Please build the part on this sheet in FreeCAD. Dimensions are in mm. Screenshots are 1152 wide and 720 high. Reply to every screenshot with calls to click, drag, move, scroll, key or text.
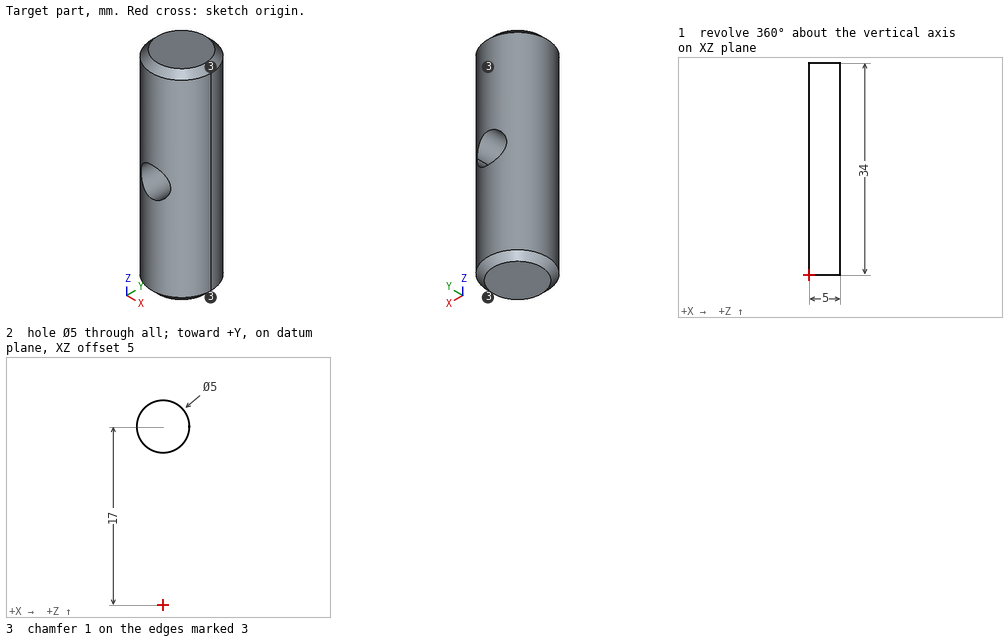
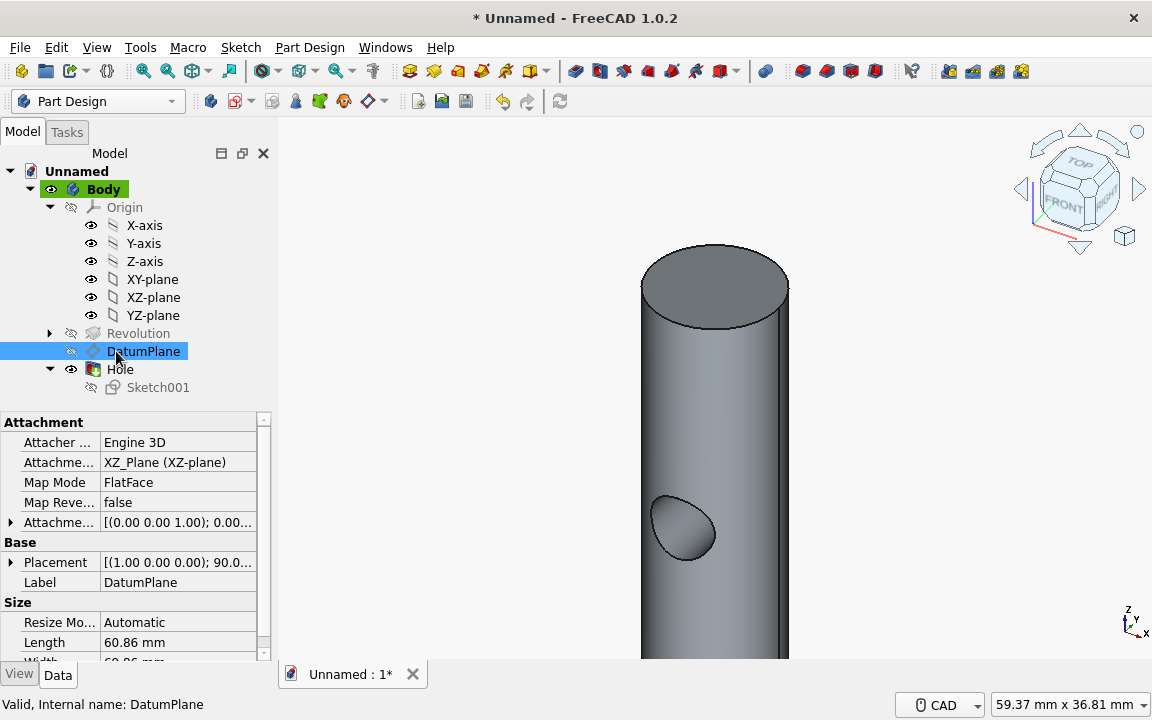
click(144, 72)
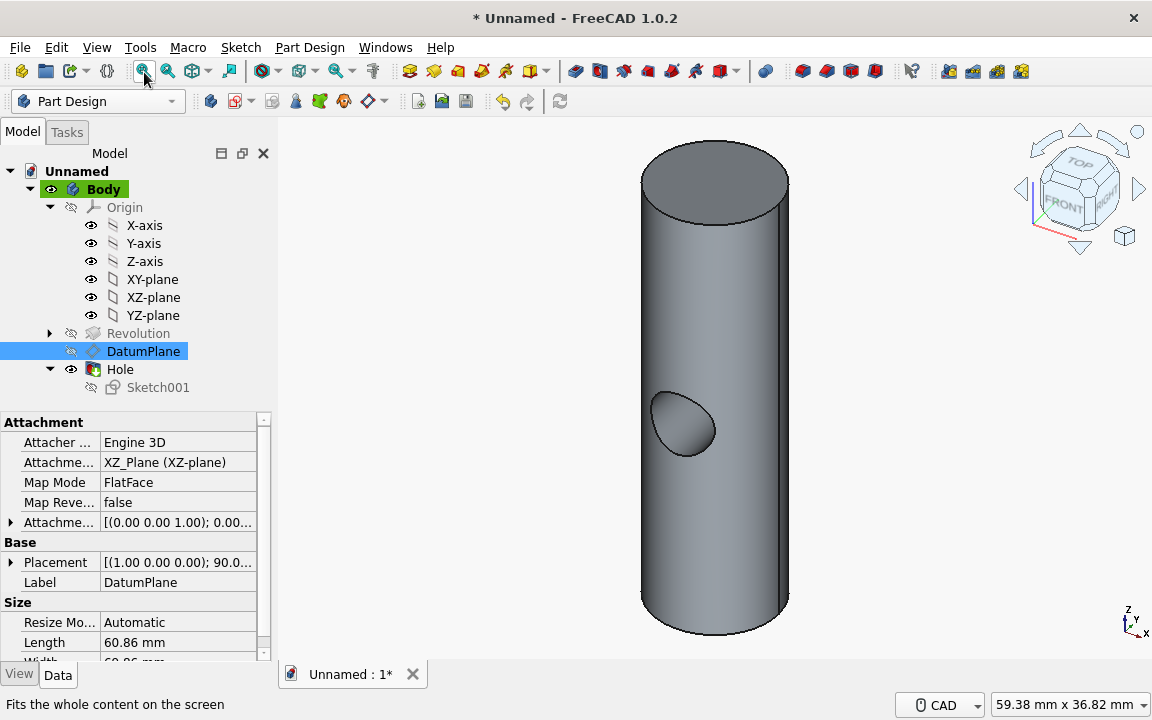
click(642, 186)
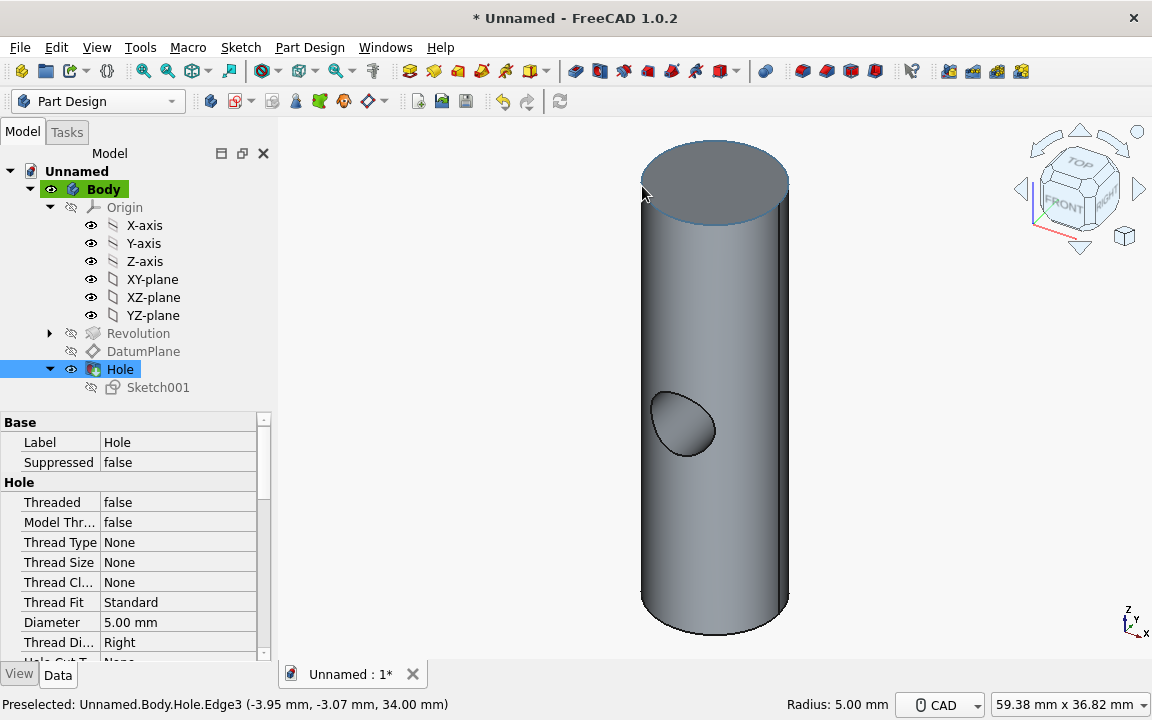
key(0)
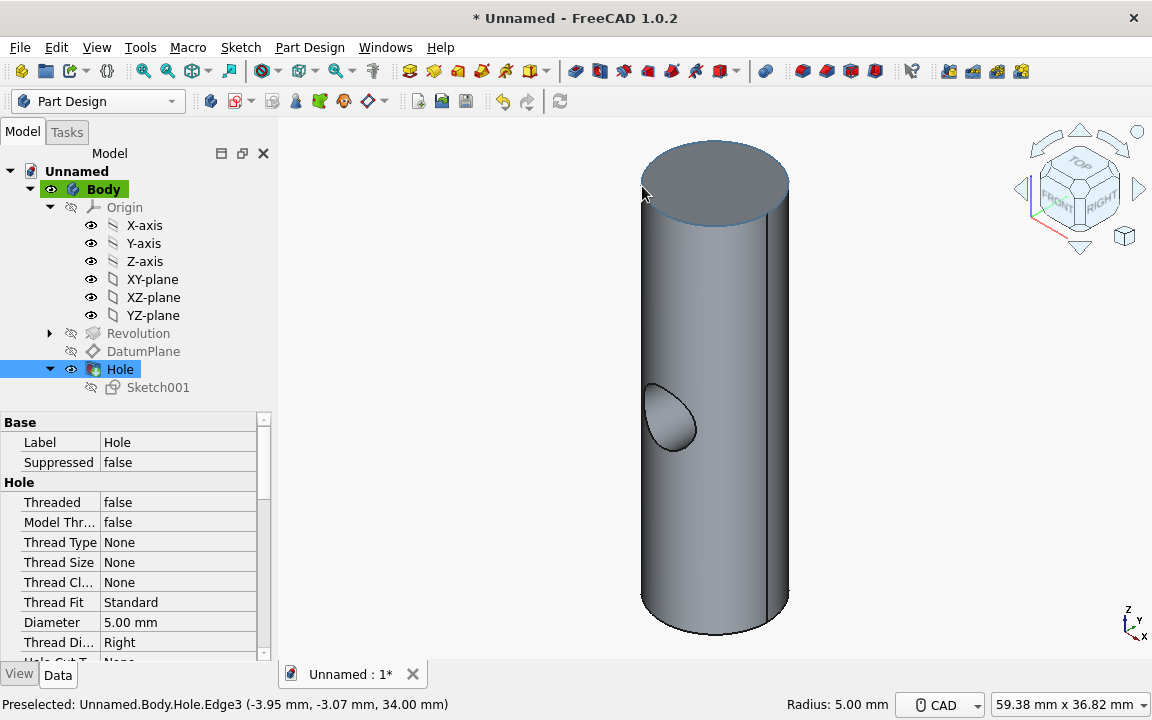
click(649, 611, ctrl)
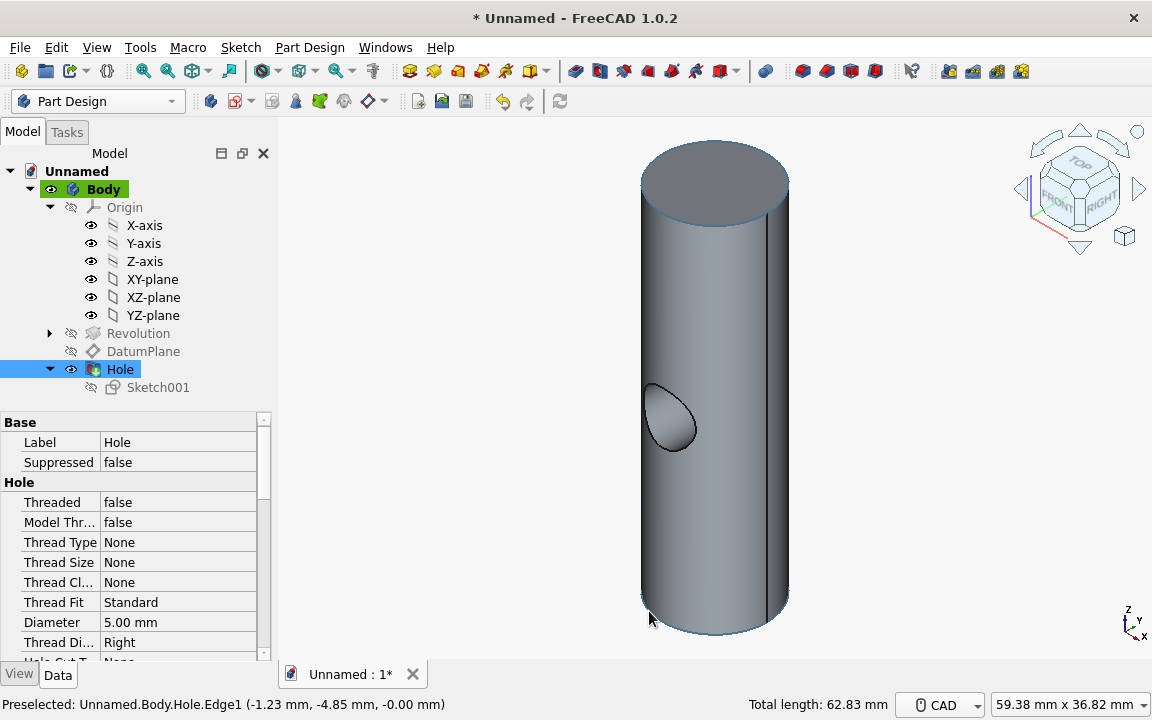
click(828, 72)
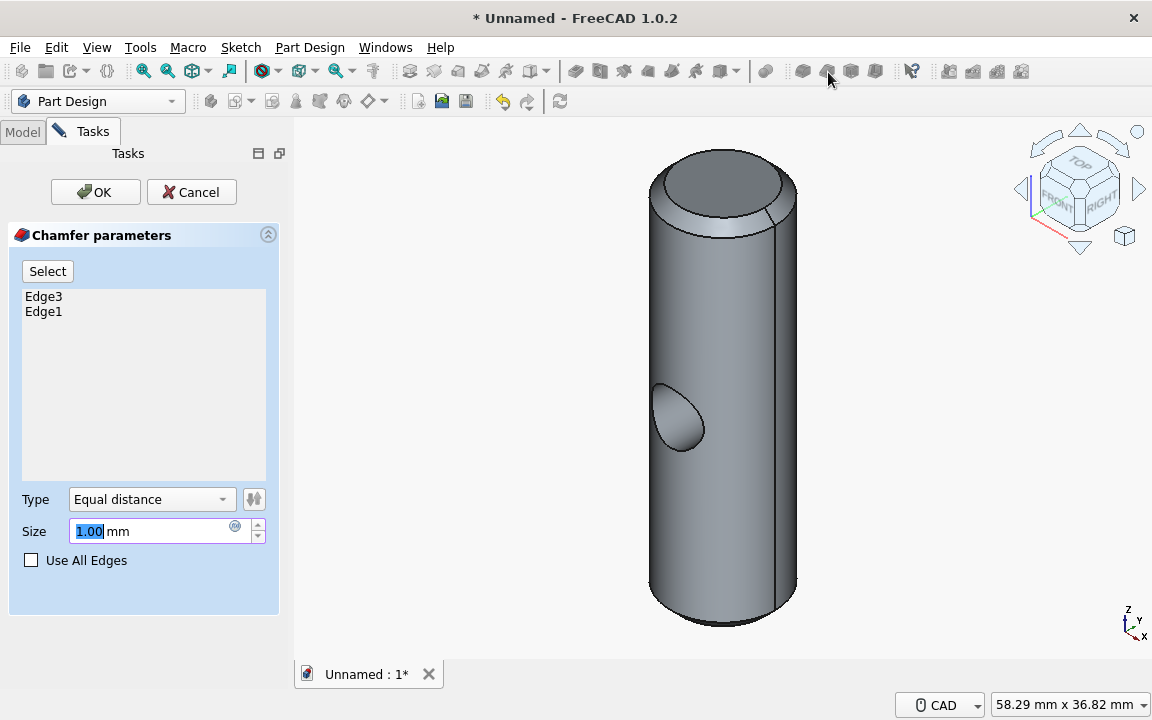
text(1)
key(Tab)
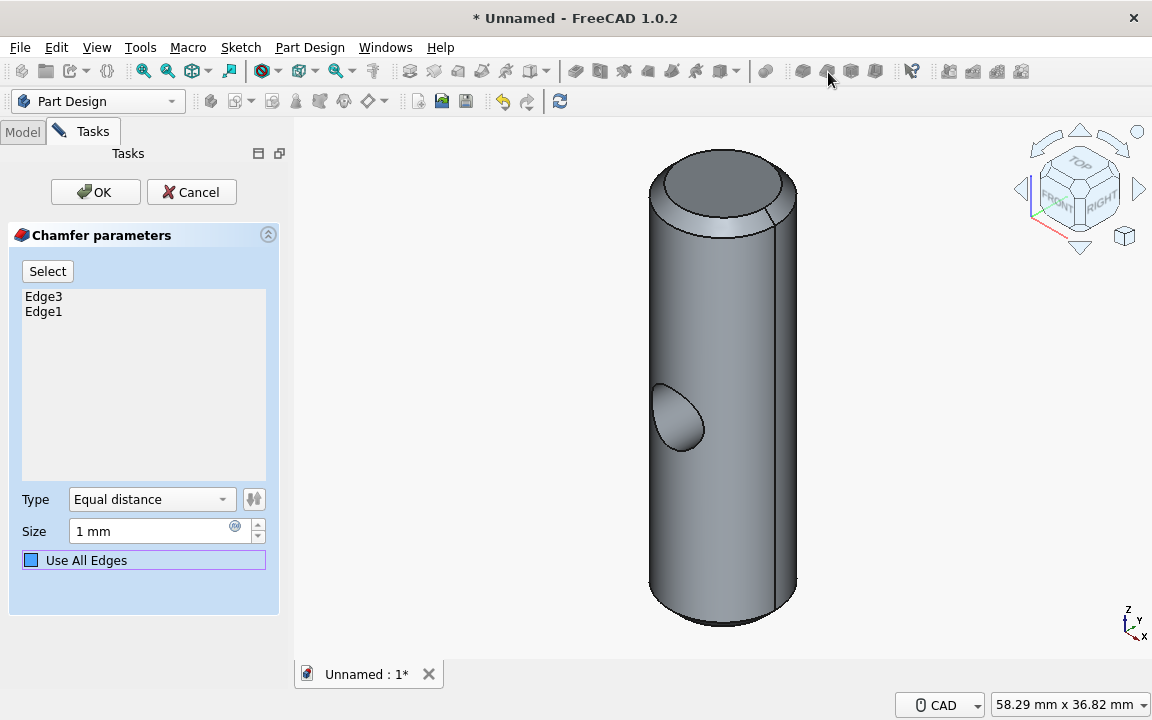
click(96, 192)